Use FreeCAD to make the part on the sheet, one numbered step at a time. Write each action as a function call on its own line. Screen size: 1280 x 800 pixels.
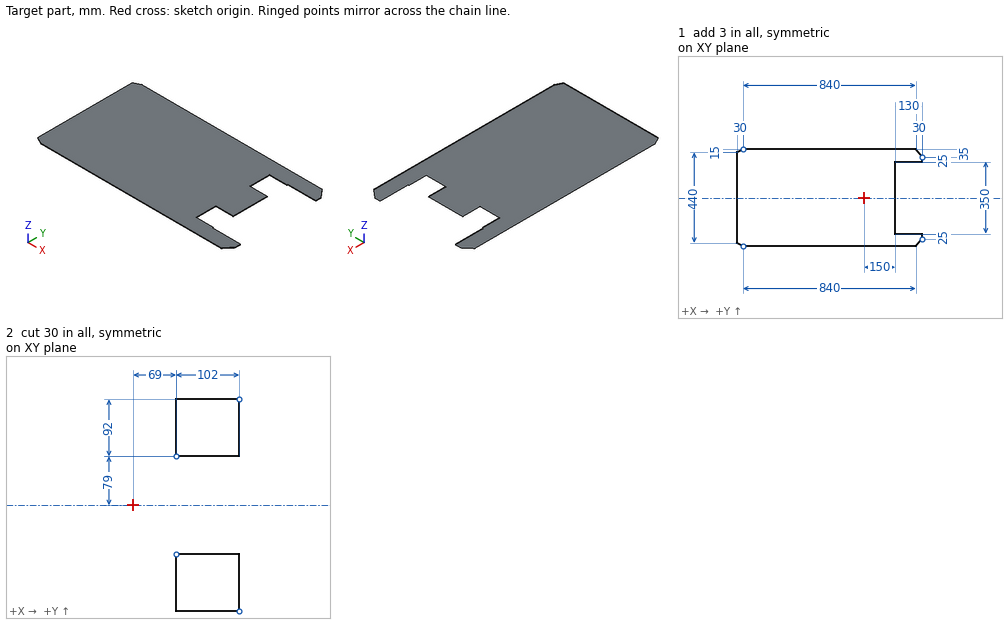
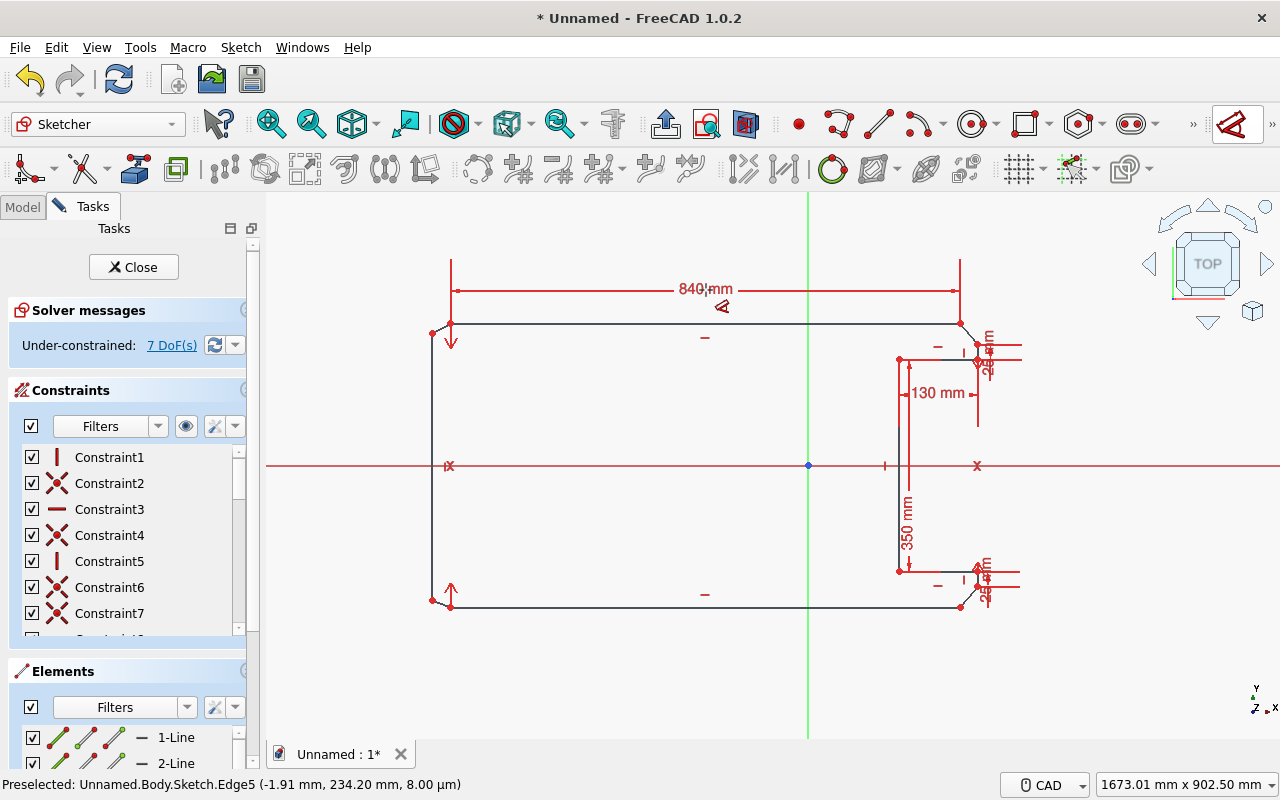
click(432, 413)
click(398, 405)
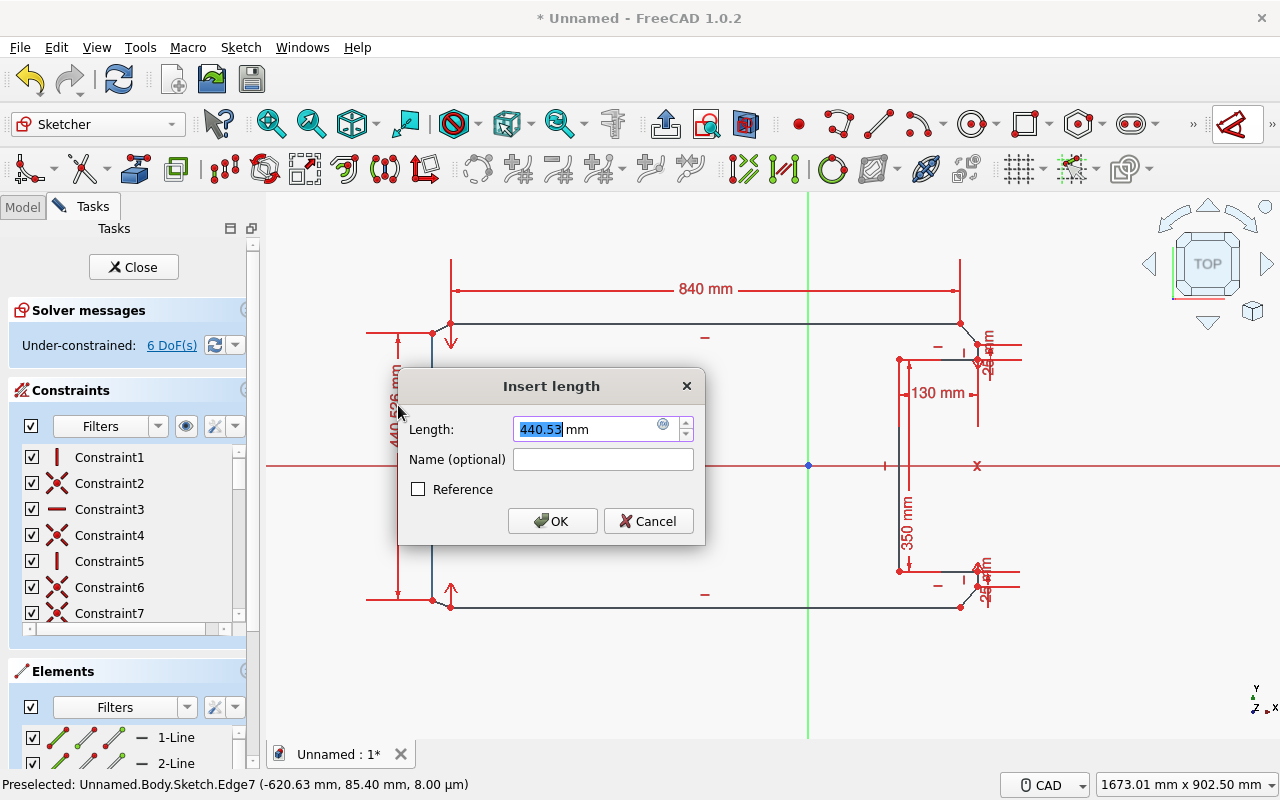
text(440)
key(Return)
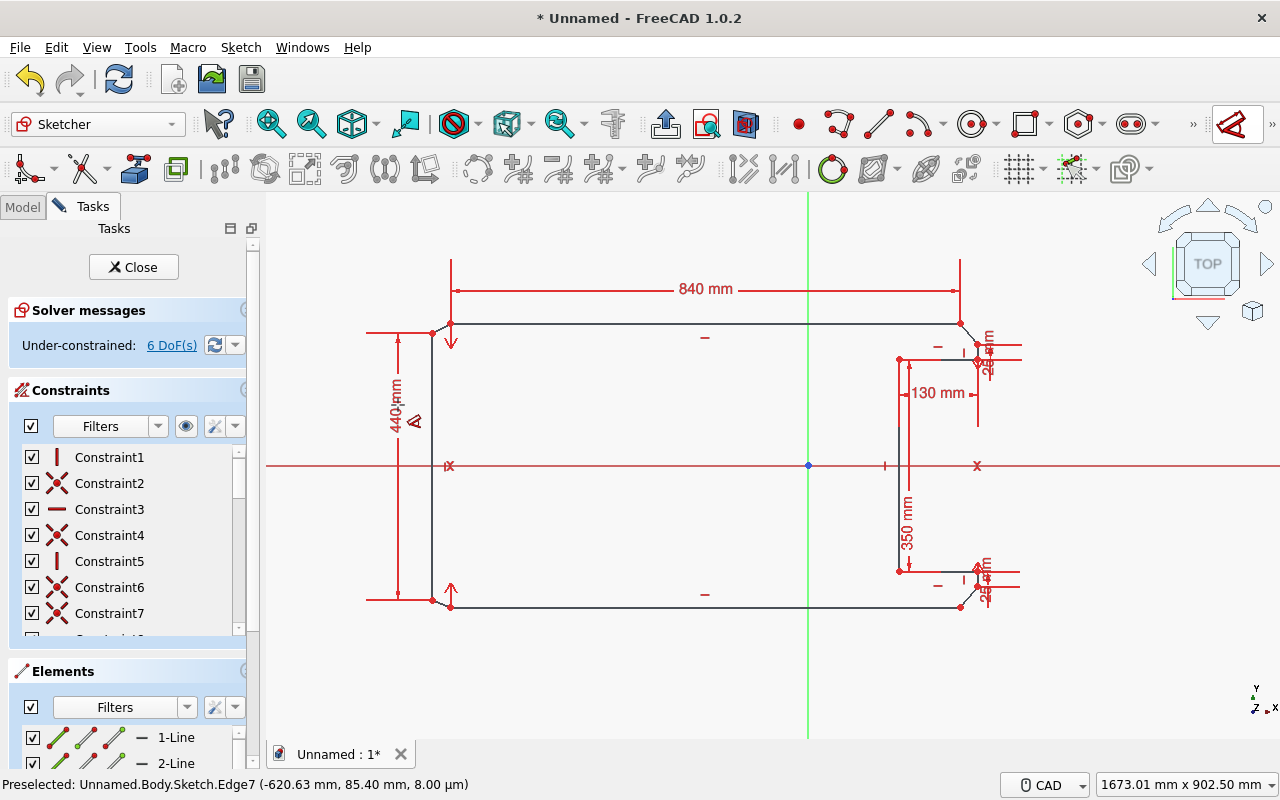
click(604, 608)
click(705, 642)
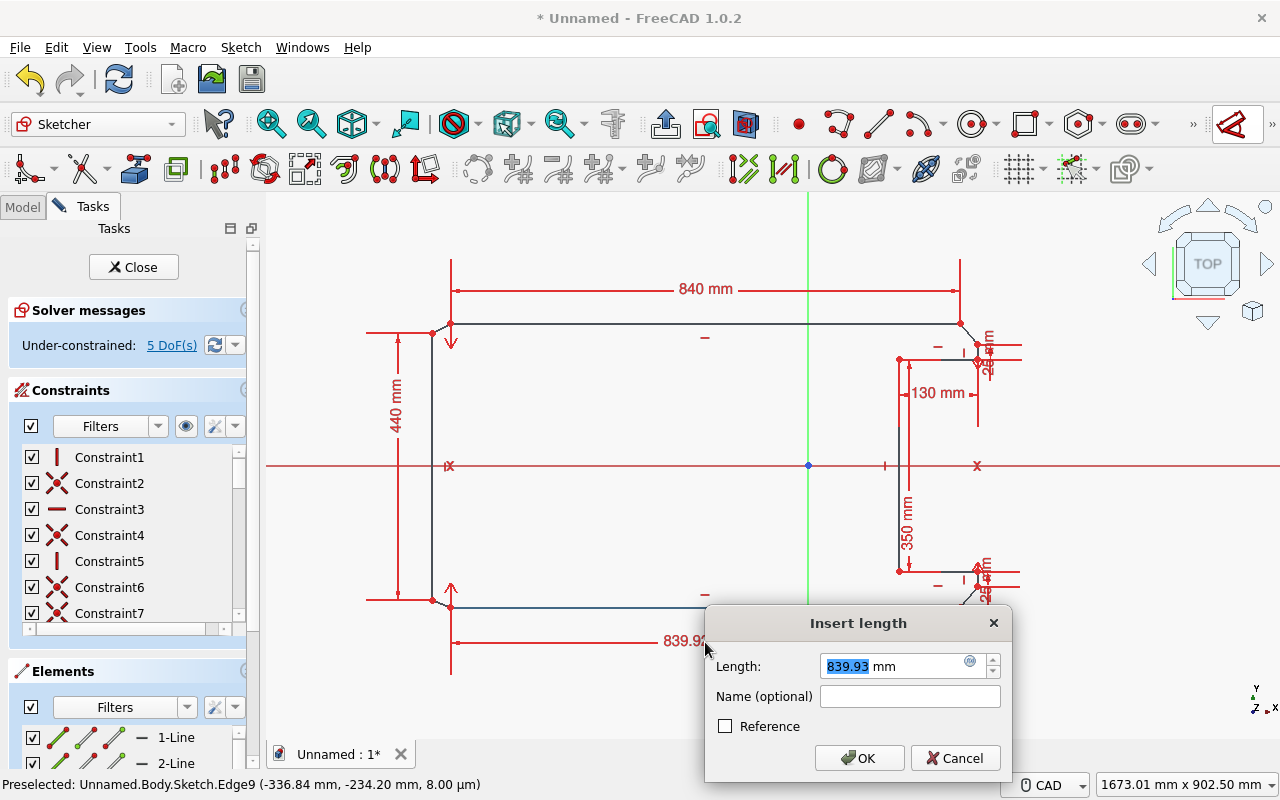
text(840)
key(Return)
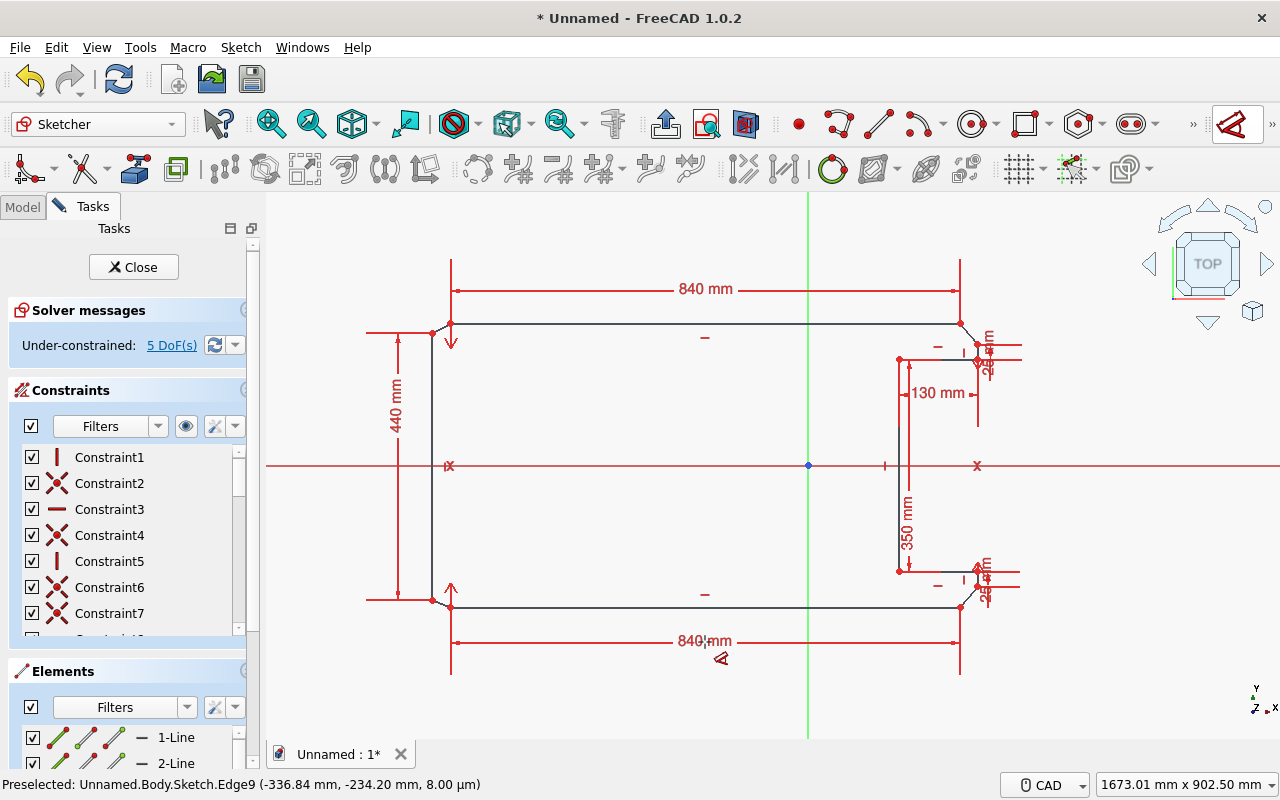
scroll(971, 336, up, 4)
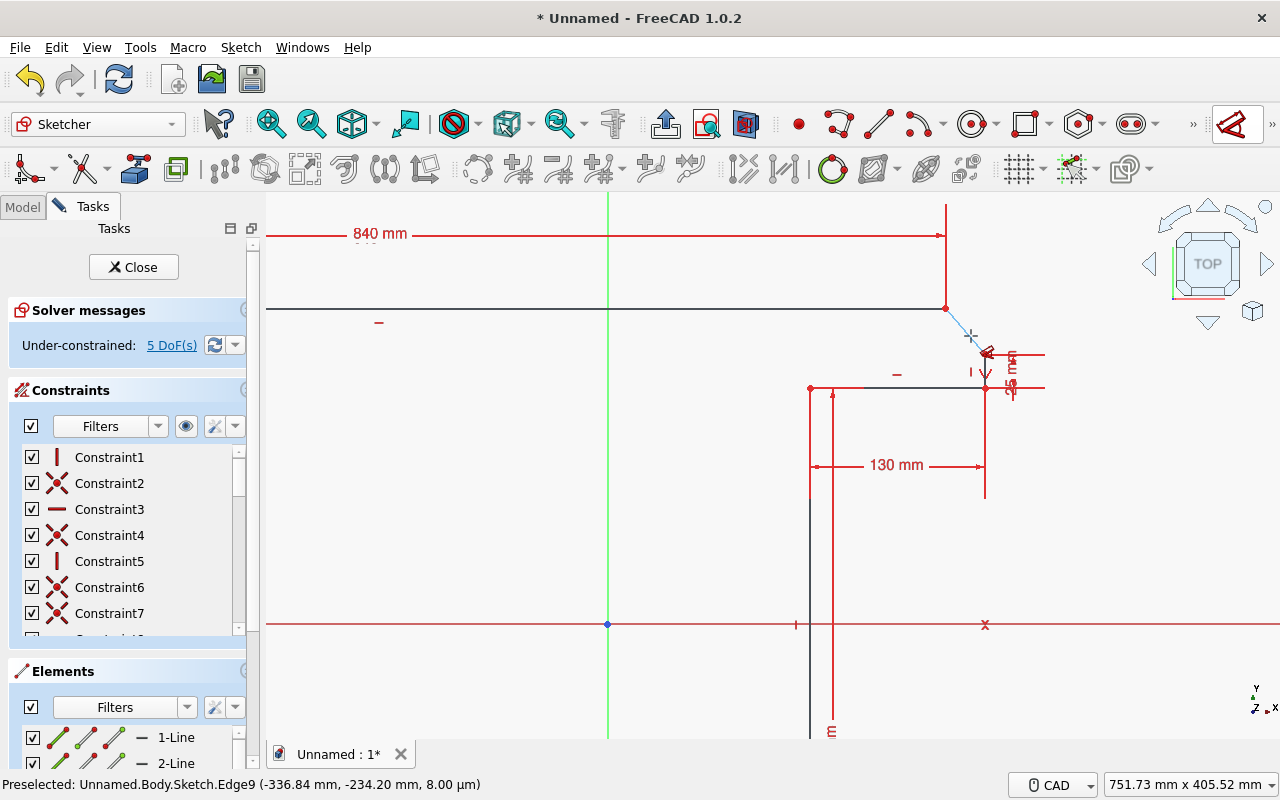
click(969, 336)
click(966, 275)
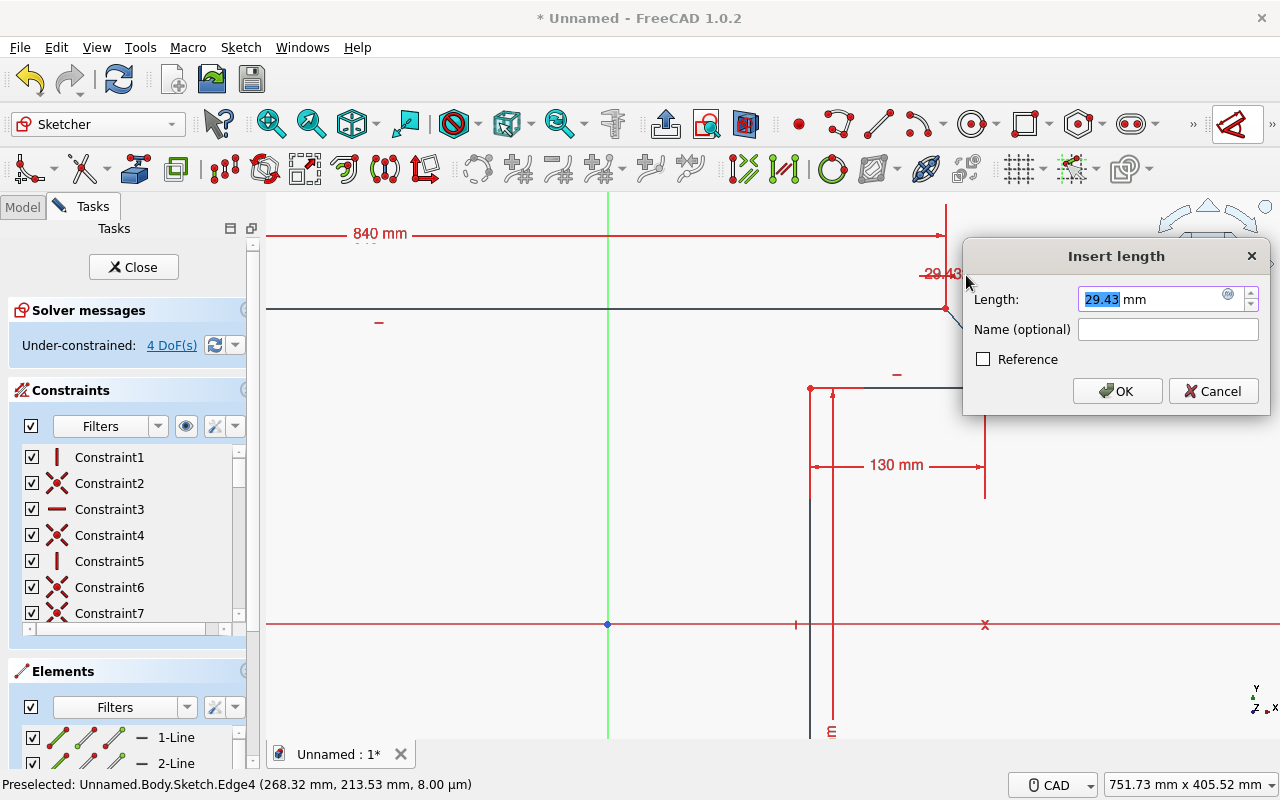
text(30)
key(Return)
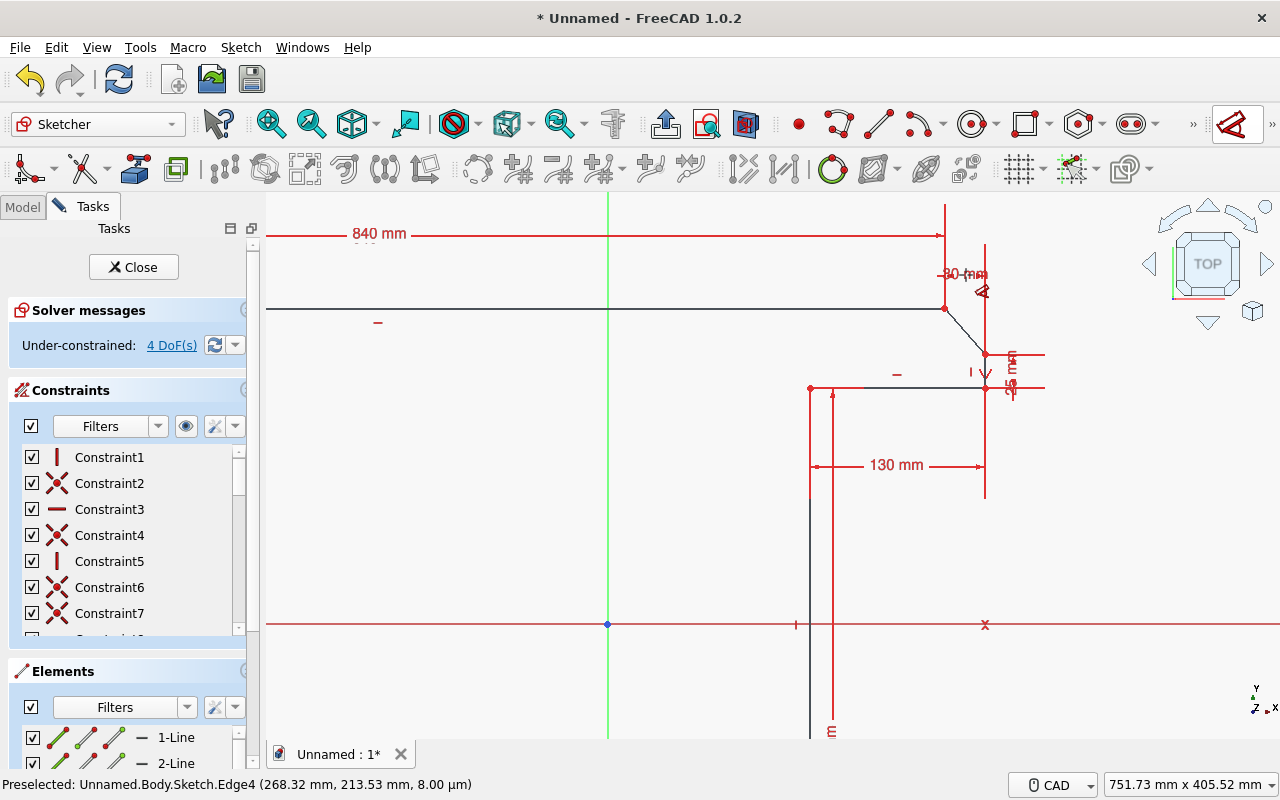
click(973, 341)
click(1019, 332)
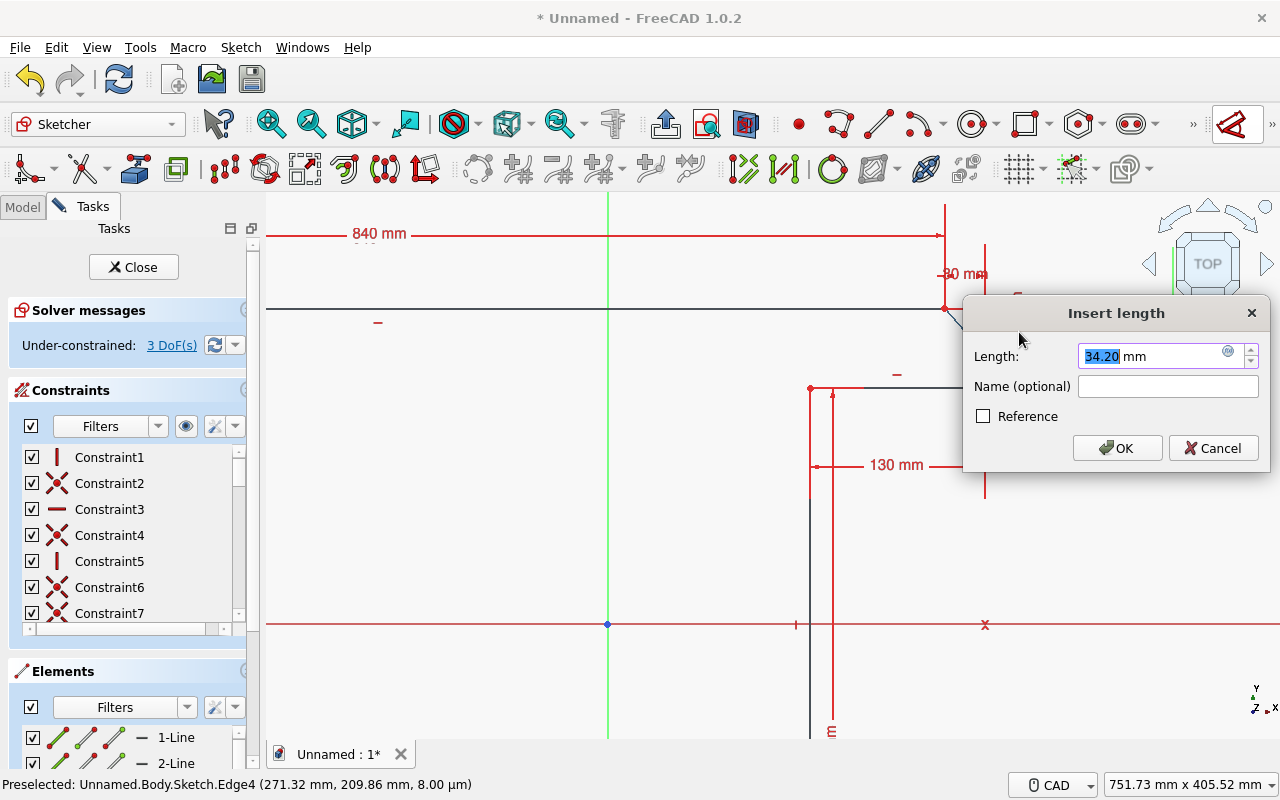
text(35)
key(Return)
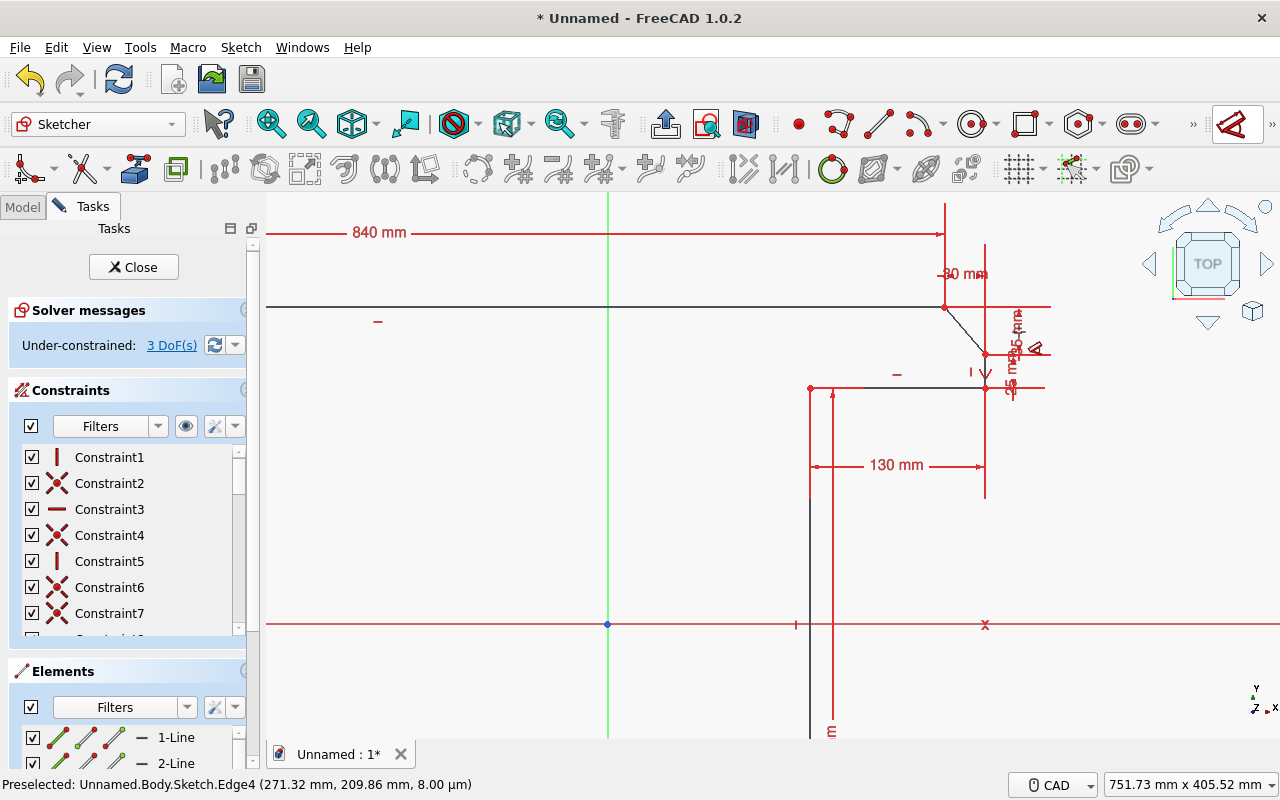
scroll(971, 336, down, 4)